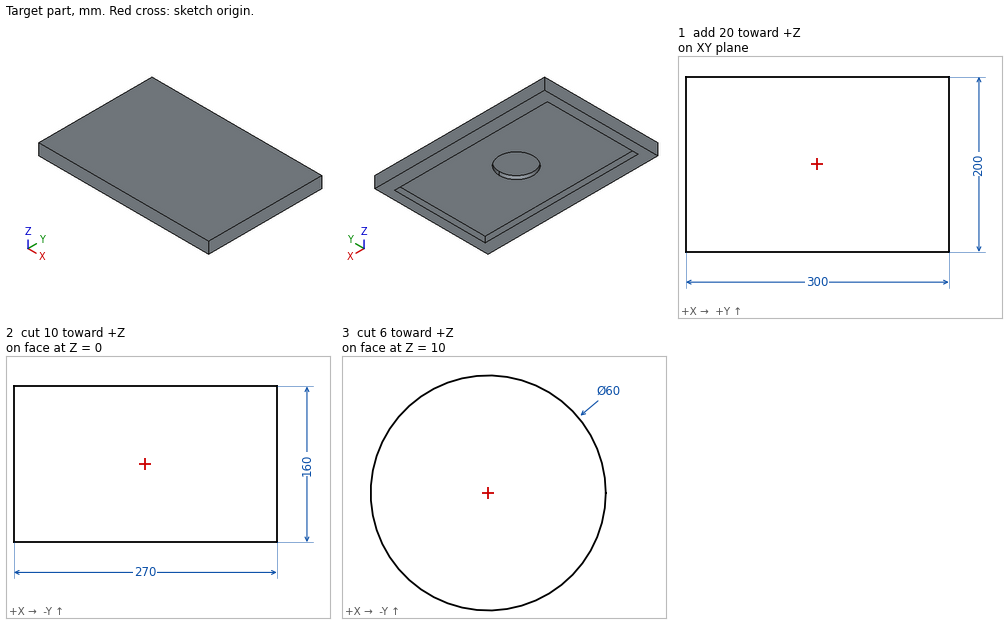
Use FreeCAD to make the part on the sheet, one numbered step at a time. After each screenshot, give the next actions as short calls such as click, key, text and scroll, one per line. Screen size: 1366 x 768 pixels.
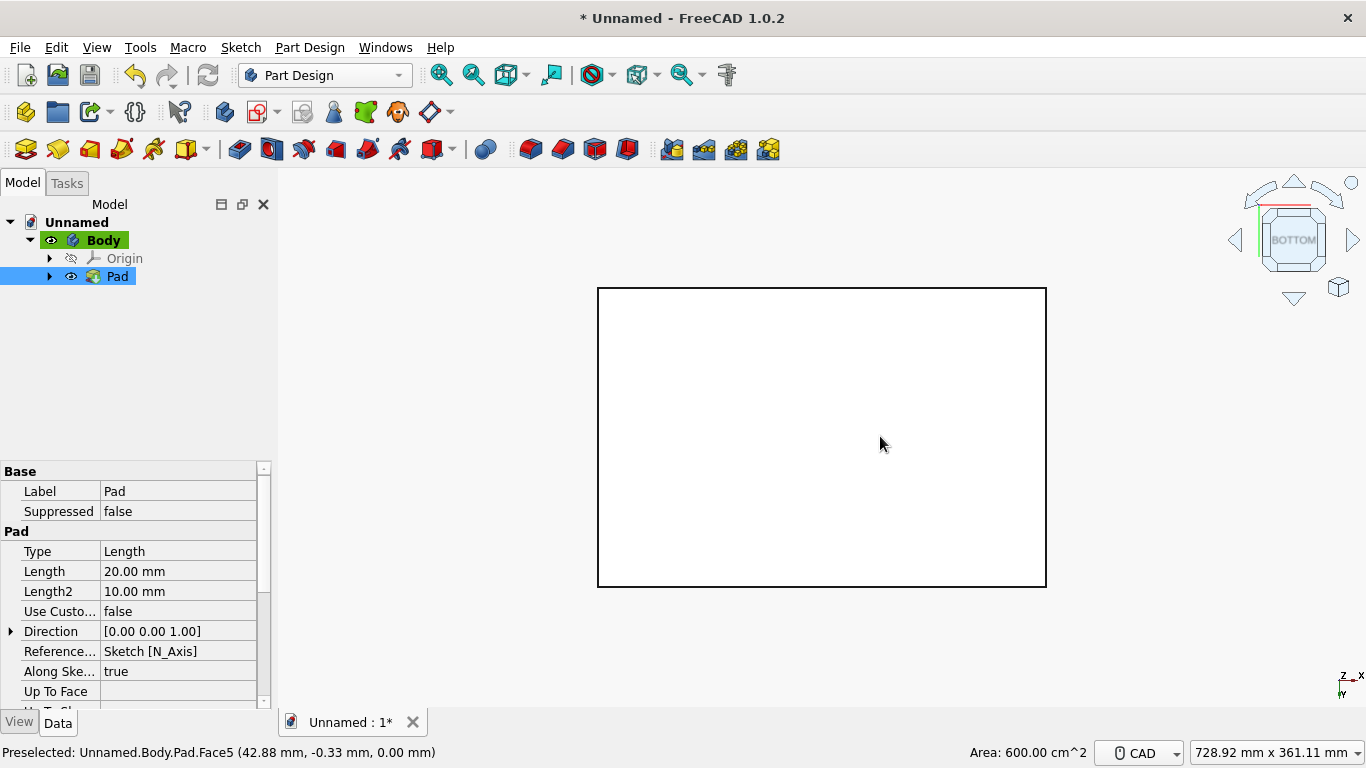
click(258, 112)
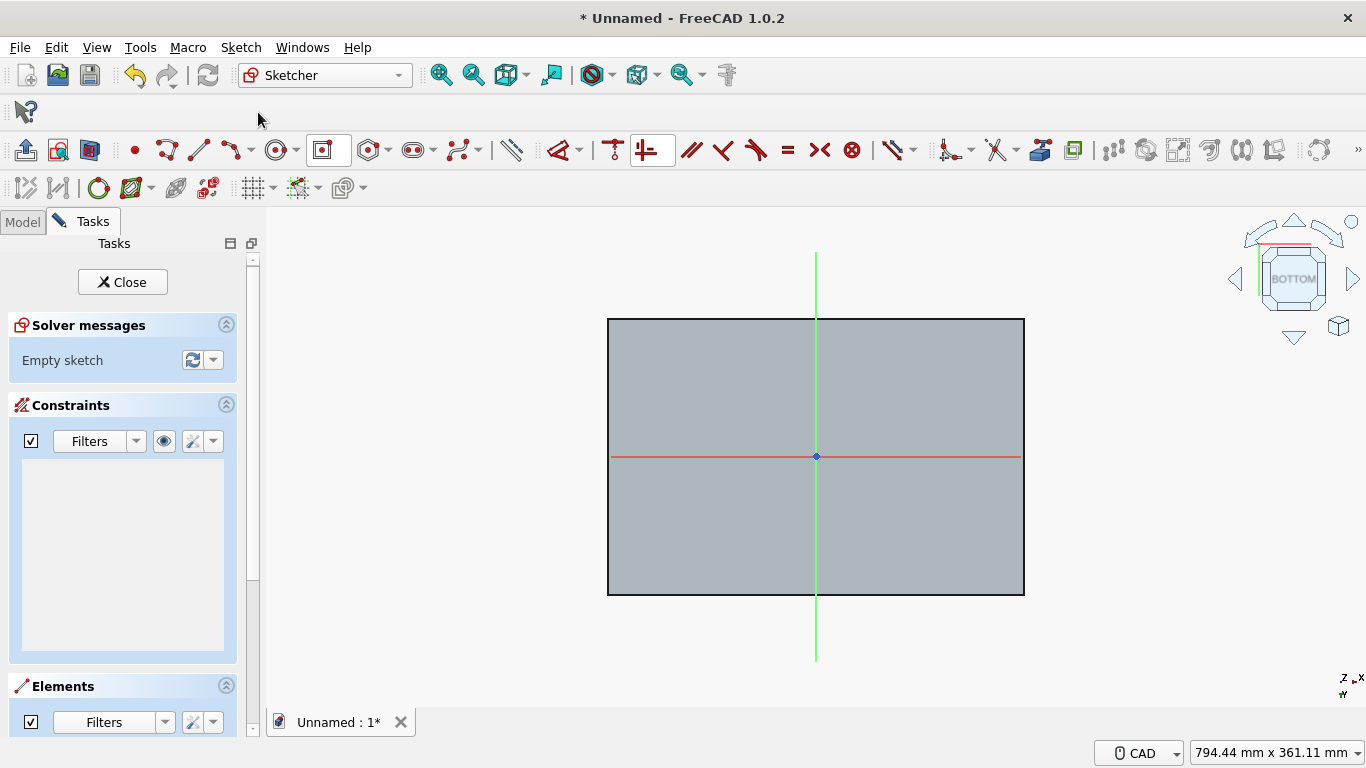
scroll(955, 457, up, 2)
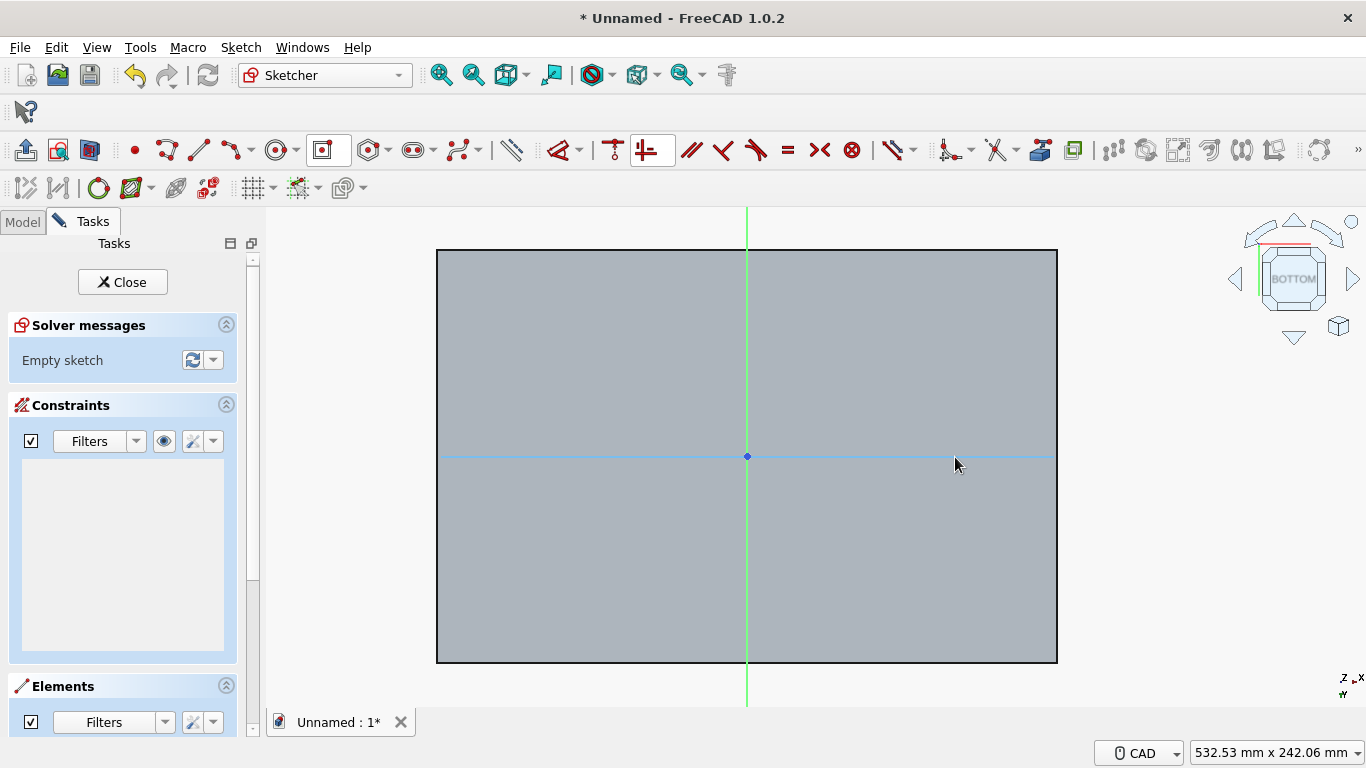
click(322, 150)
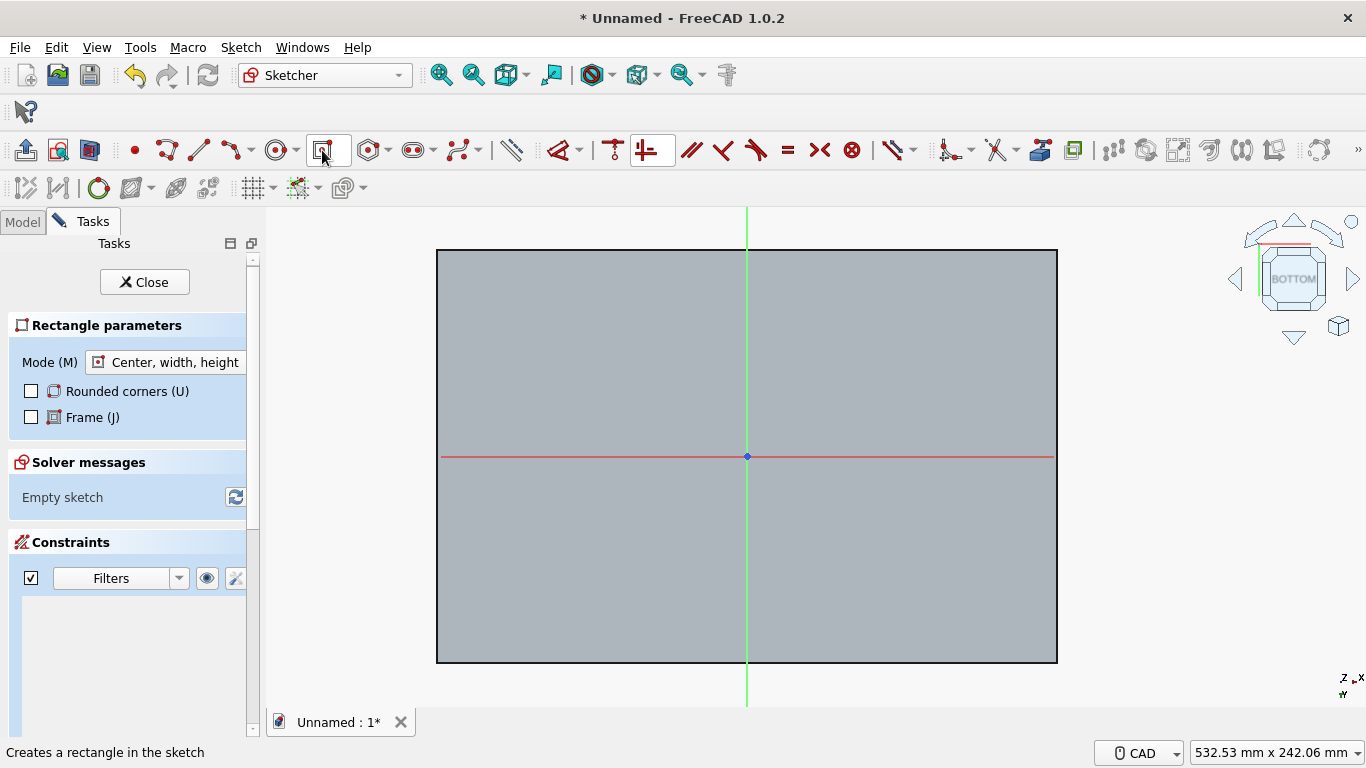
click(747, 457)
click(1026, 292)
key(Escape)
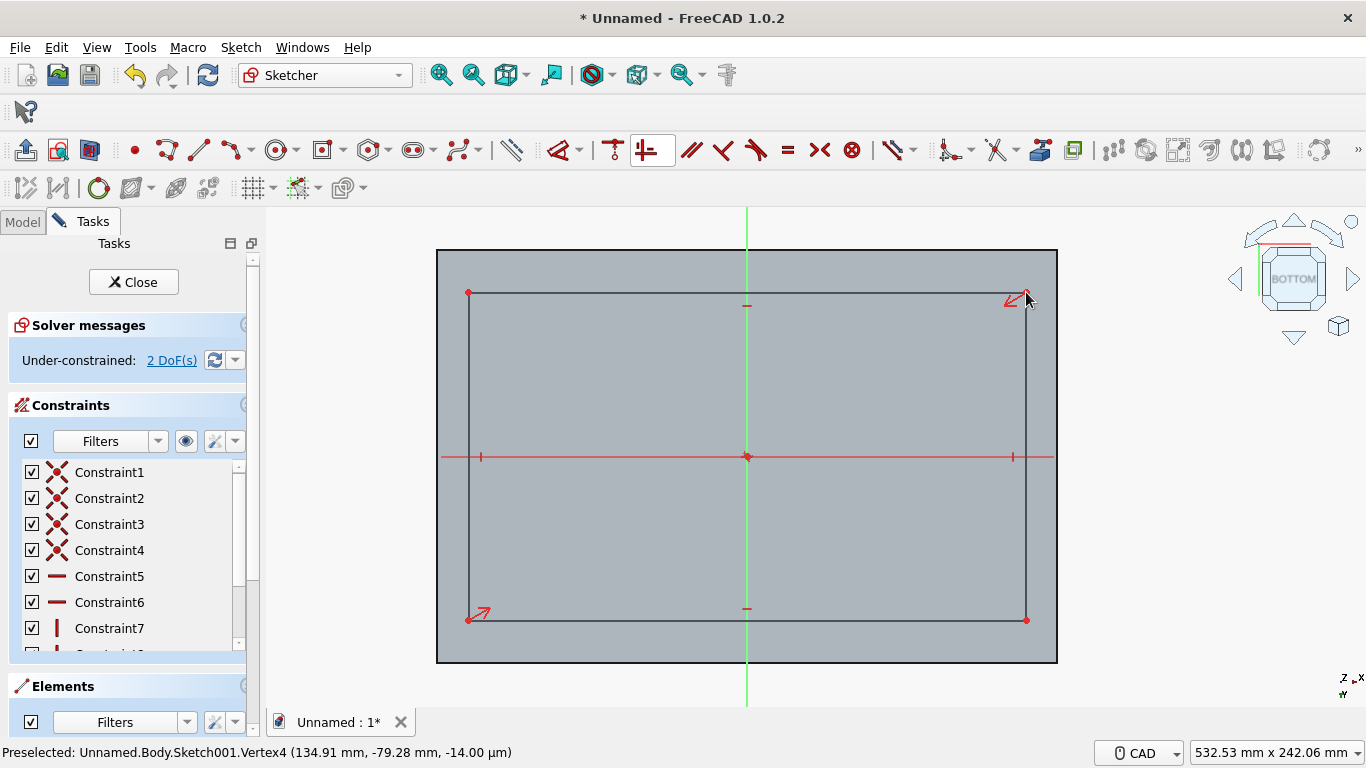
click(636, 621)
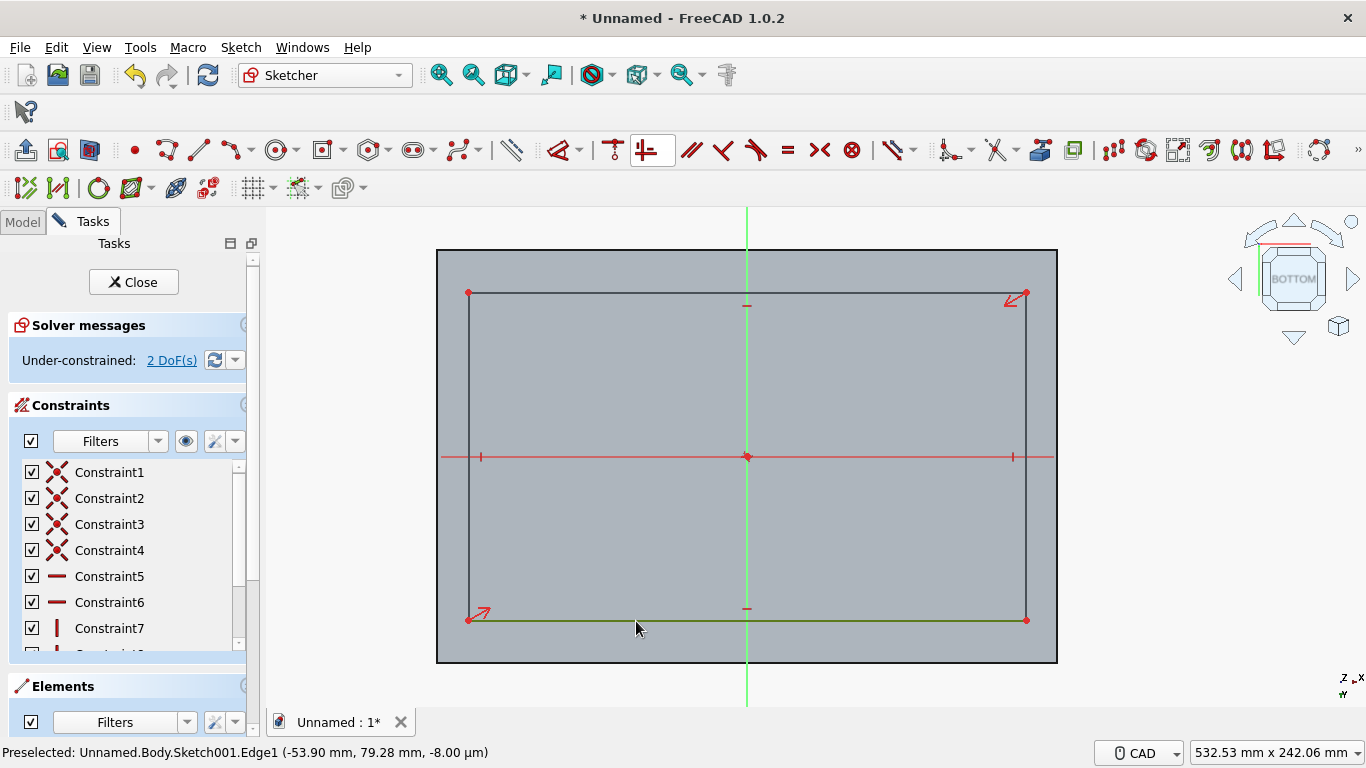
key(l)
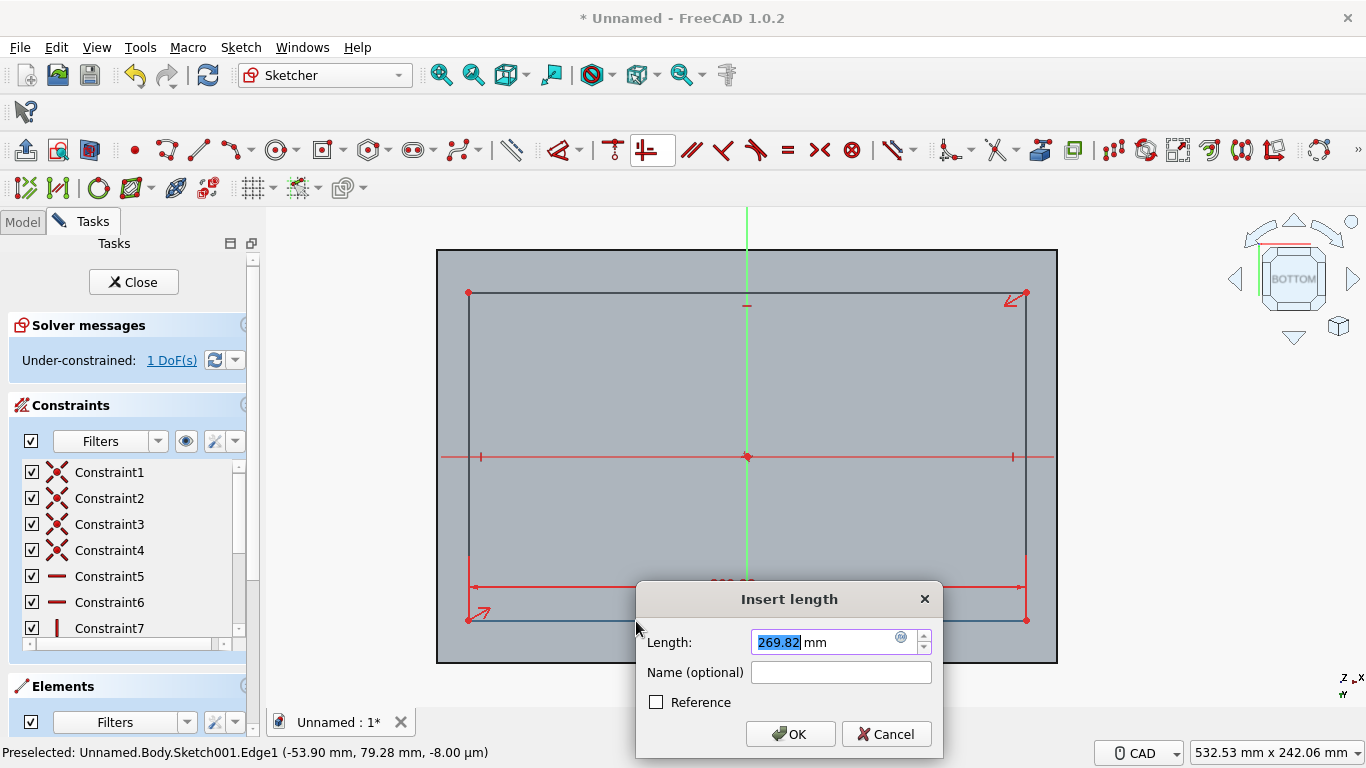
text(270)
key(Return)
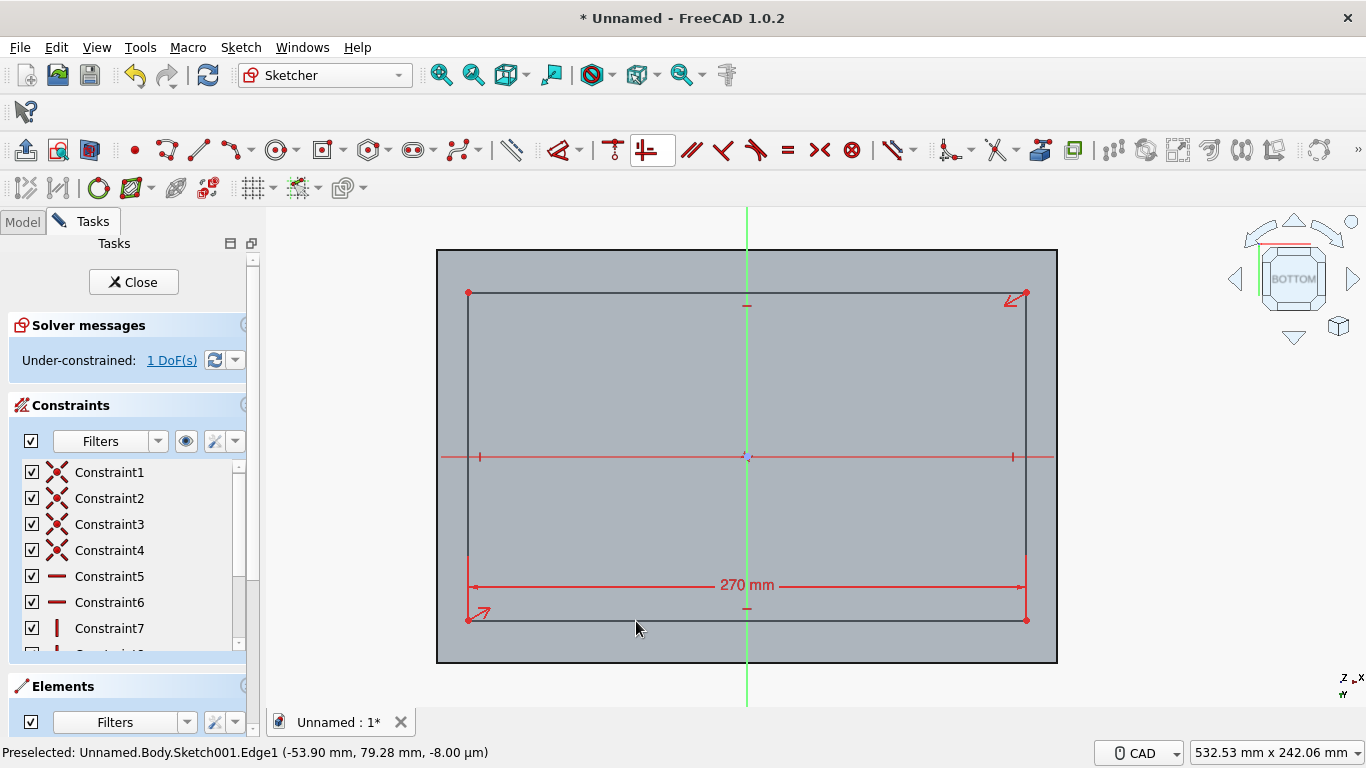
click(1026, 522)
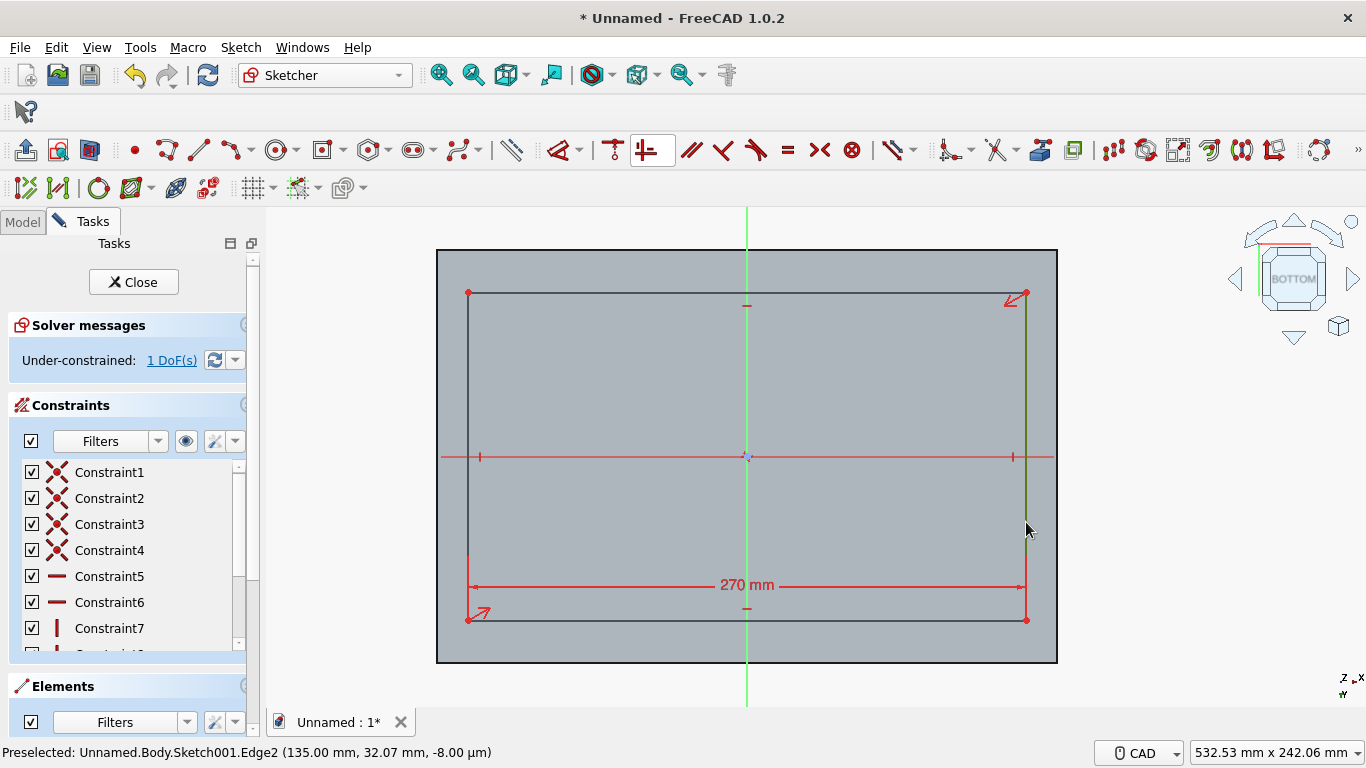
click(582, 150)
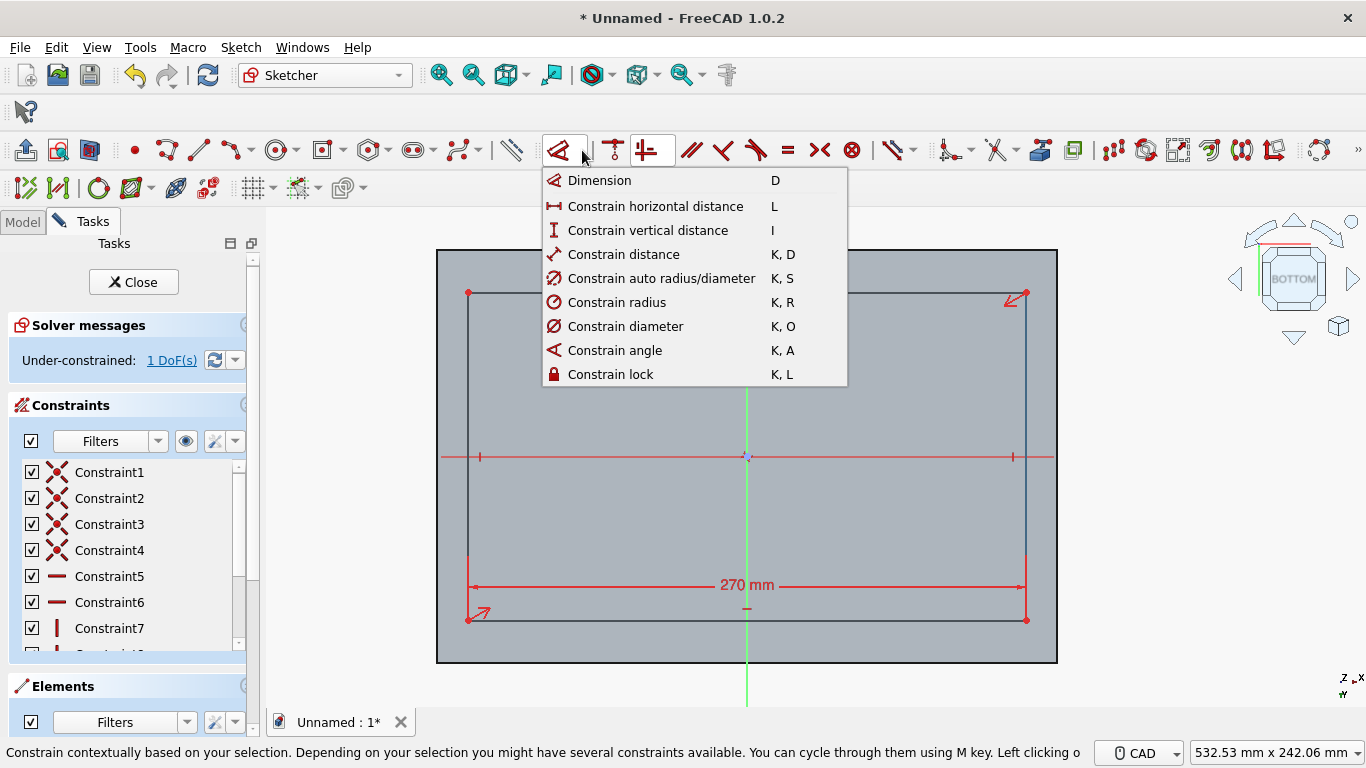
click(695, 230)